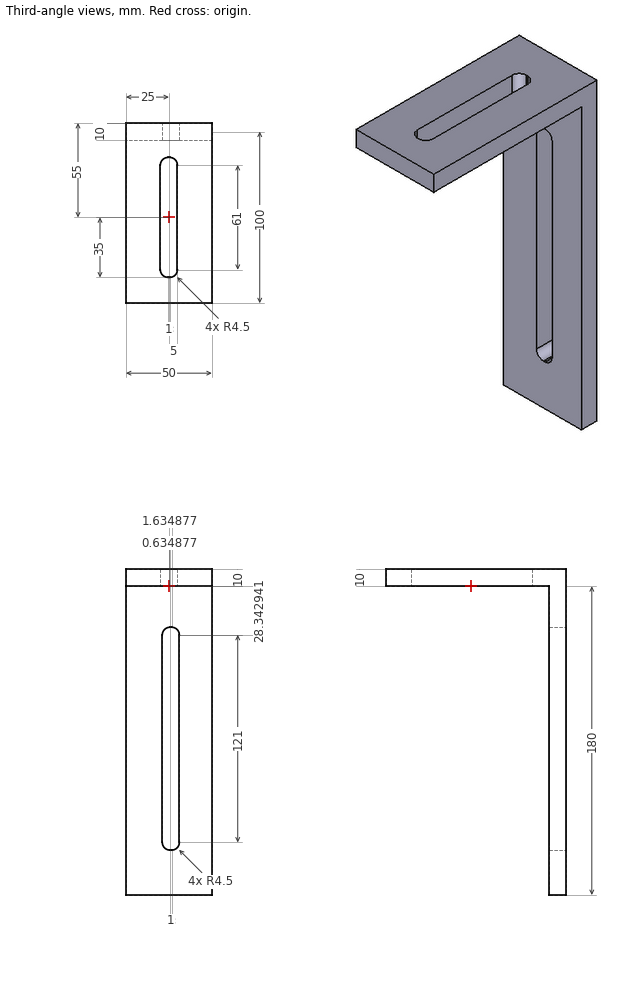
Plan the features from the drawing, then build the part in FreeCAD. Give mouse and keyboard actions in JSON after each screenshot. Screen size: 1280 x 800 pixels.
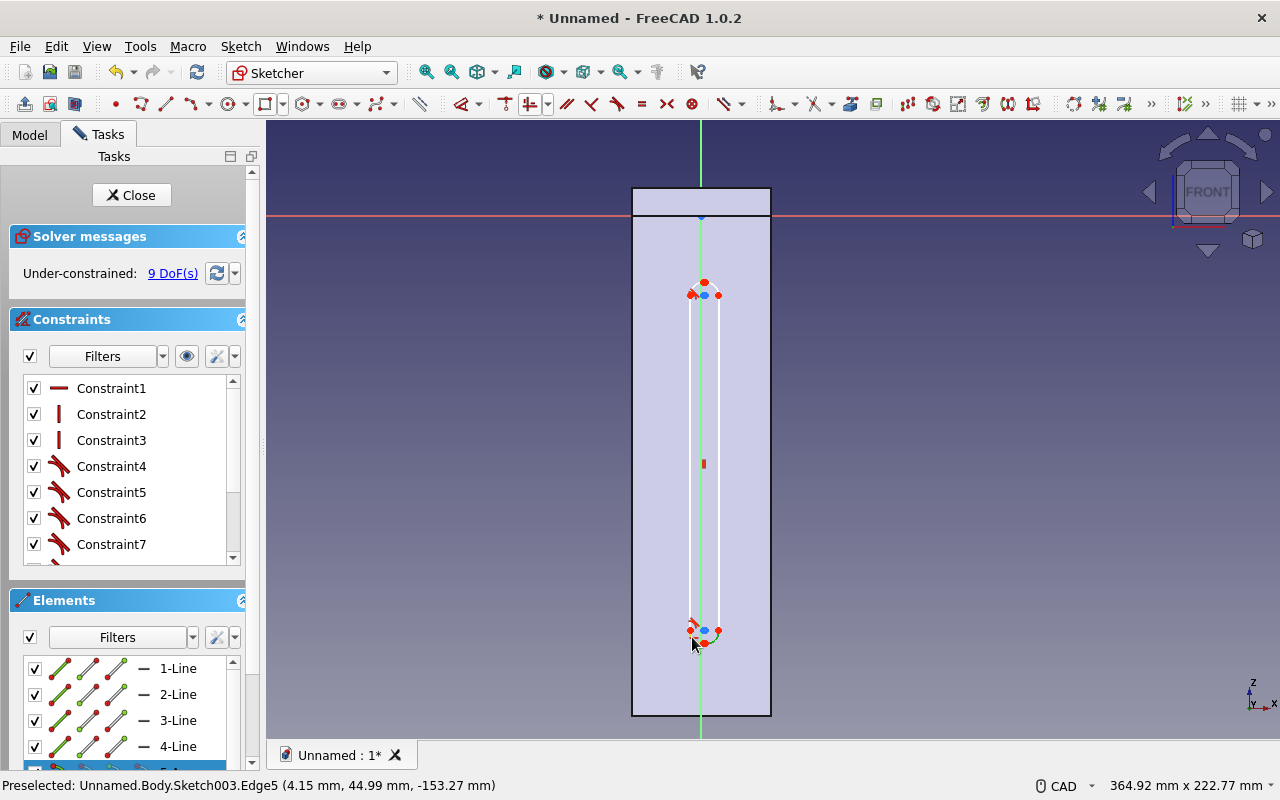
{"action": "scroll", "coordinate": [718, 290], "scroll_direction": "up", "scroll_amount": 5}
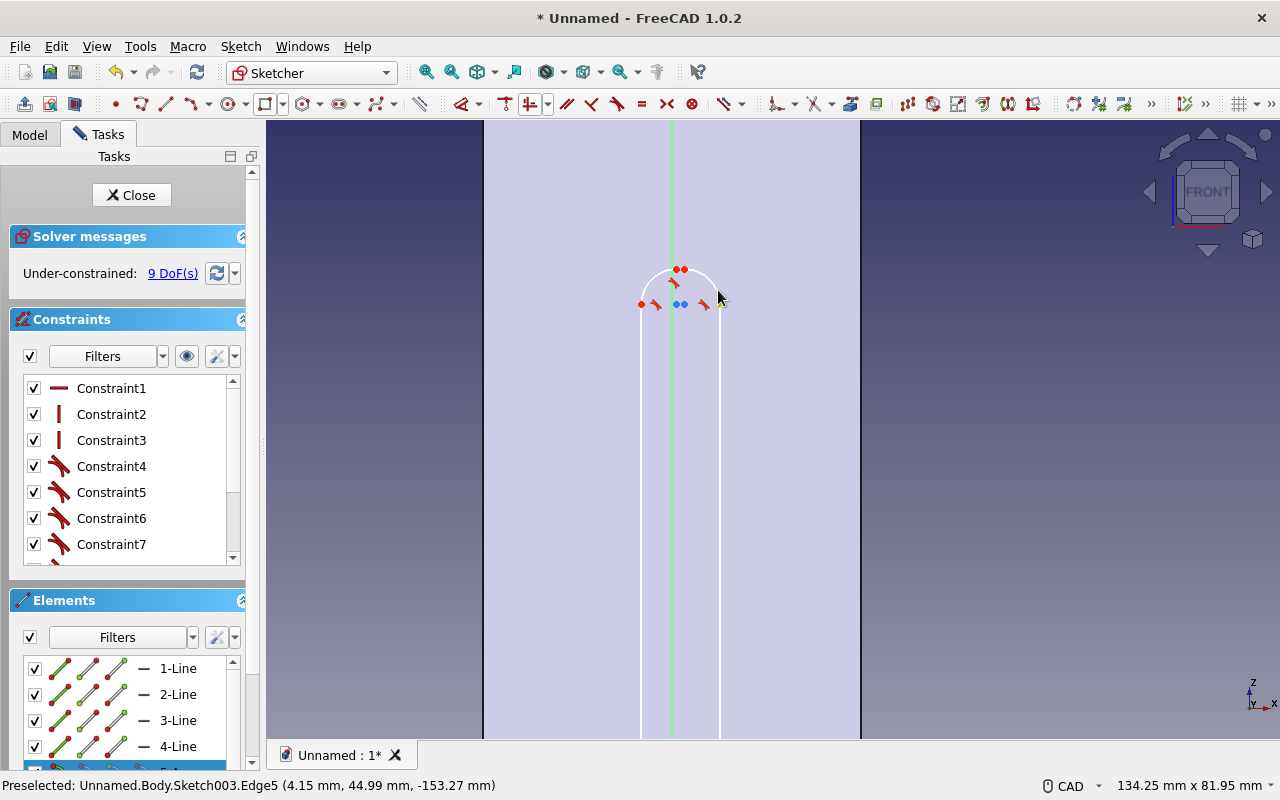
{"action": "left_click", "coordinate": [716, 288]}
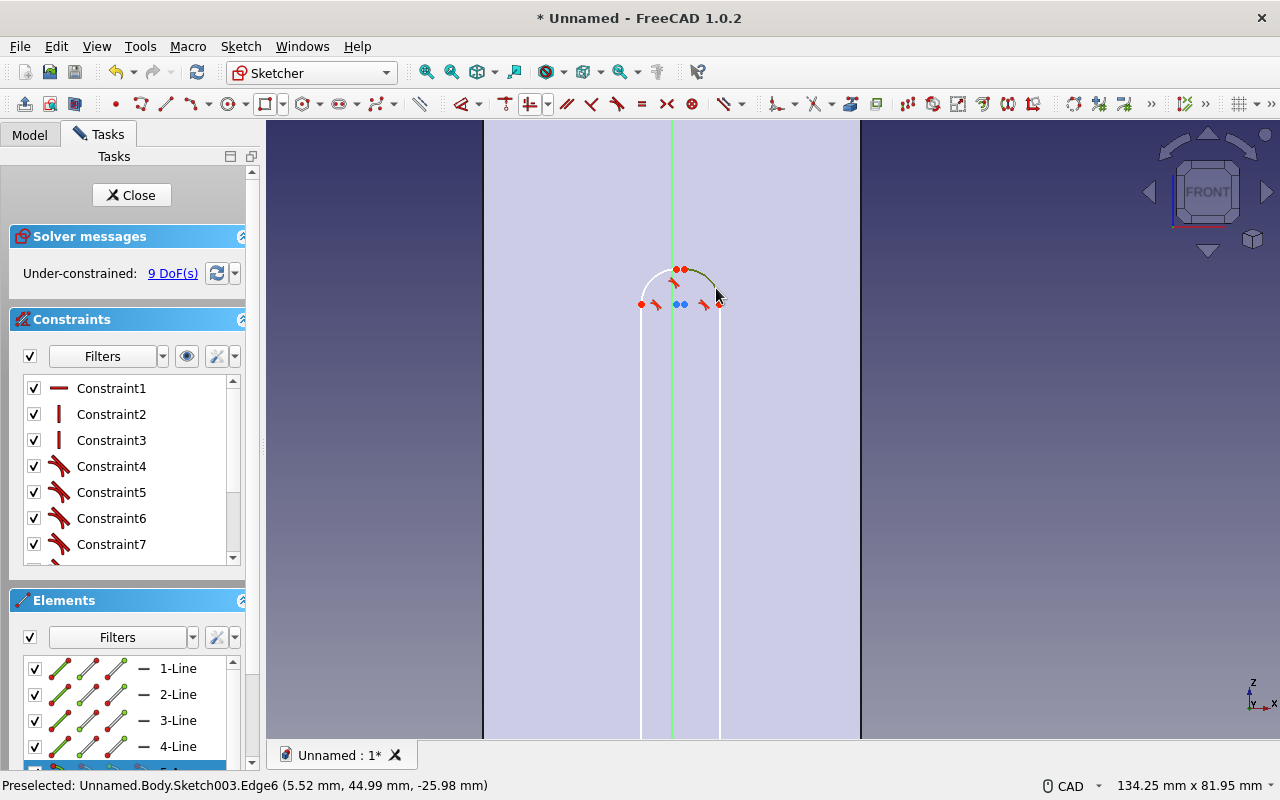
{"action": "scroll", "coordinate": [661, 273], "scroll_direction": "up", "scroll_amount": 2}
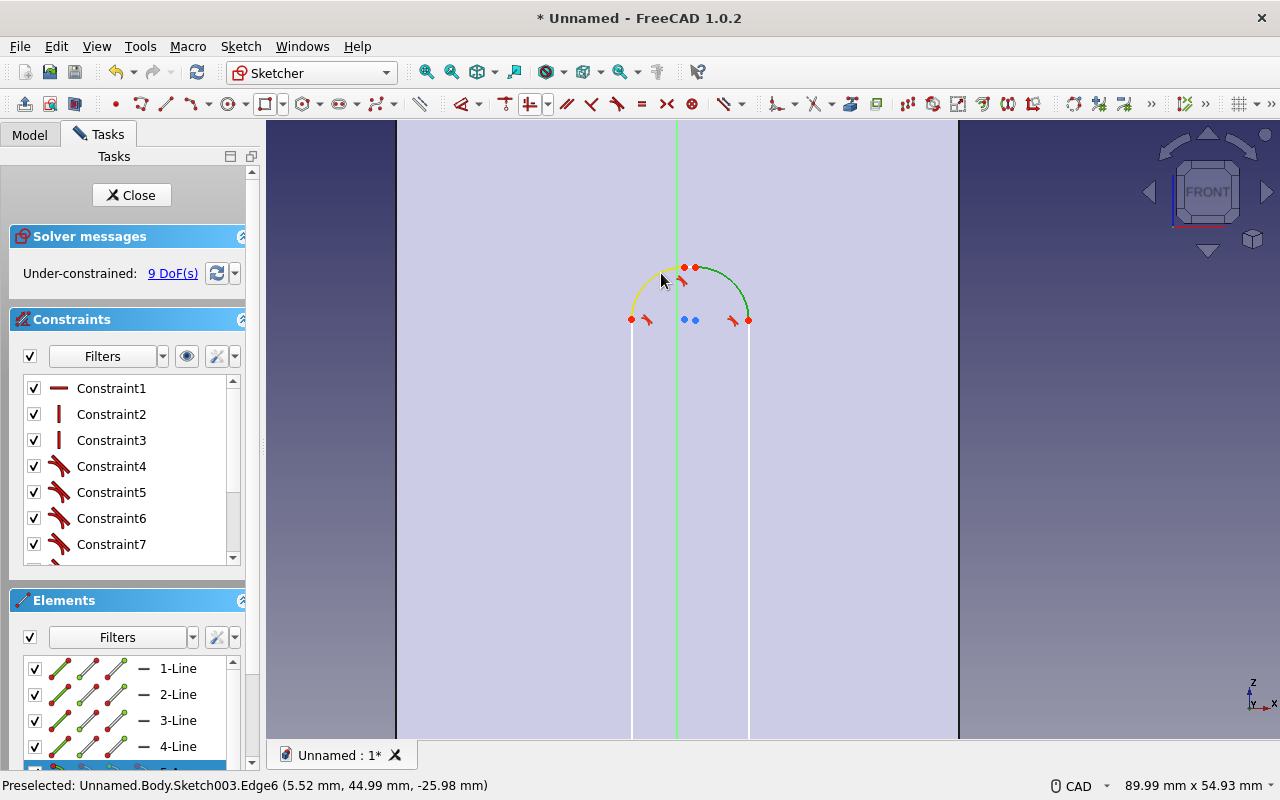
{"action": "left_click", "coordinate": [660, 273]}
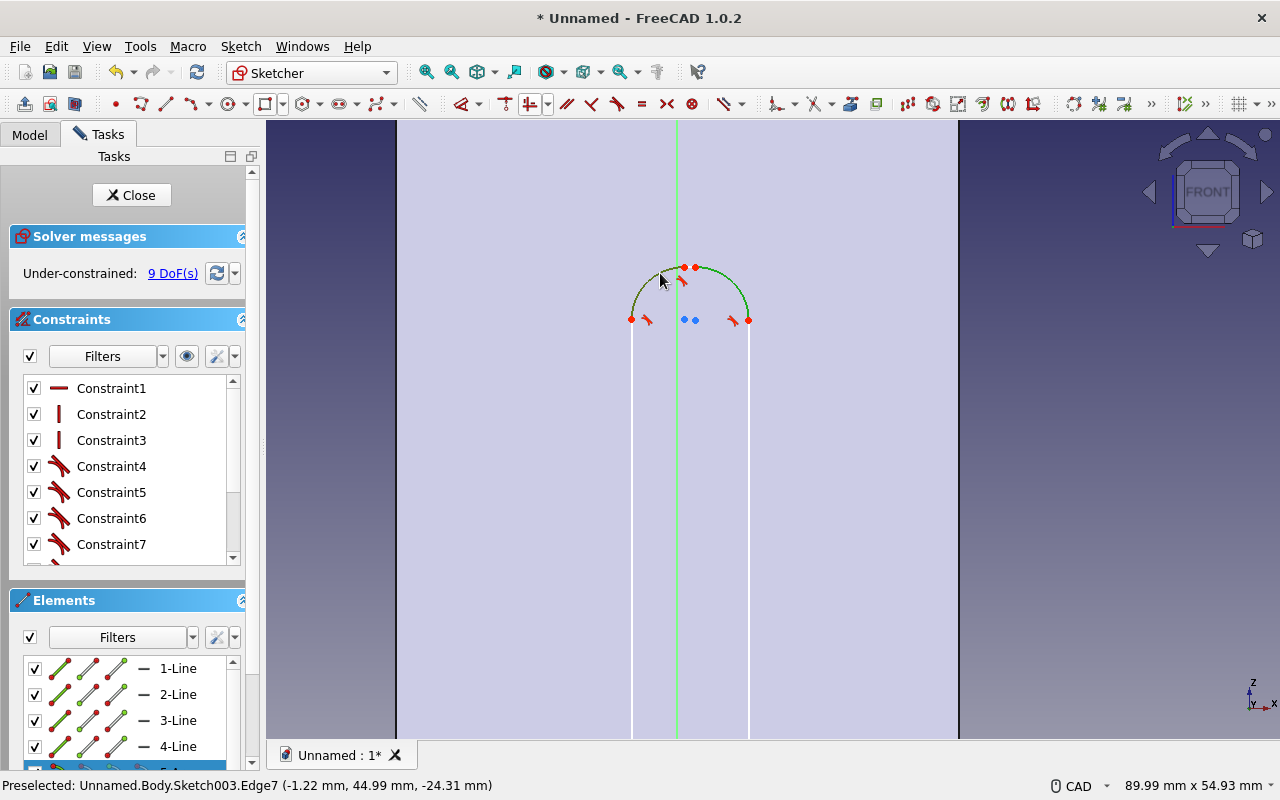
{"action": "scroll", "coordinate": [709, 287], "scroll_direction": "down", "scroll_amount": 7}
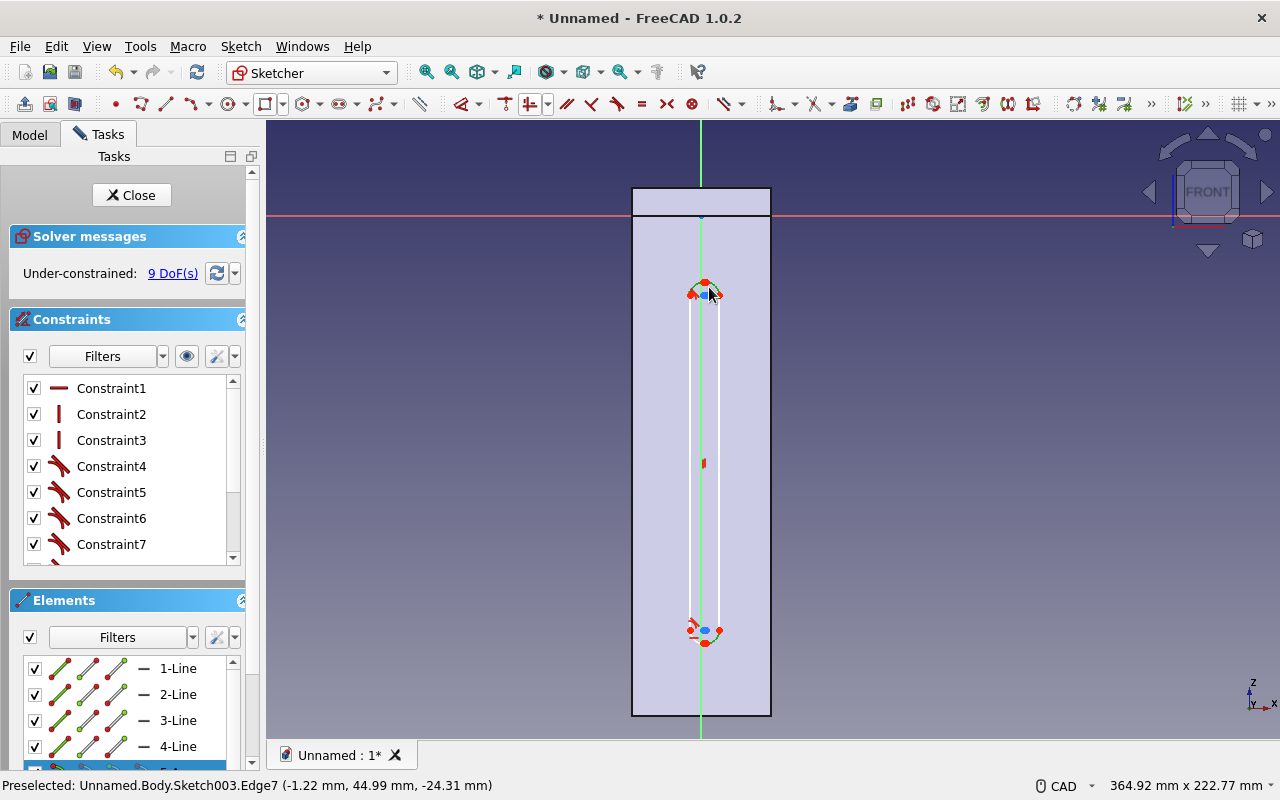
{"action": "scroll", "coordinate": [692, 636], "scroll_direction": "up", "scroll_amount": 4}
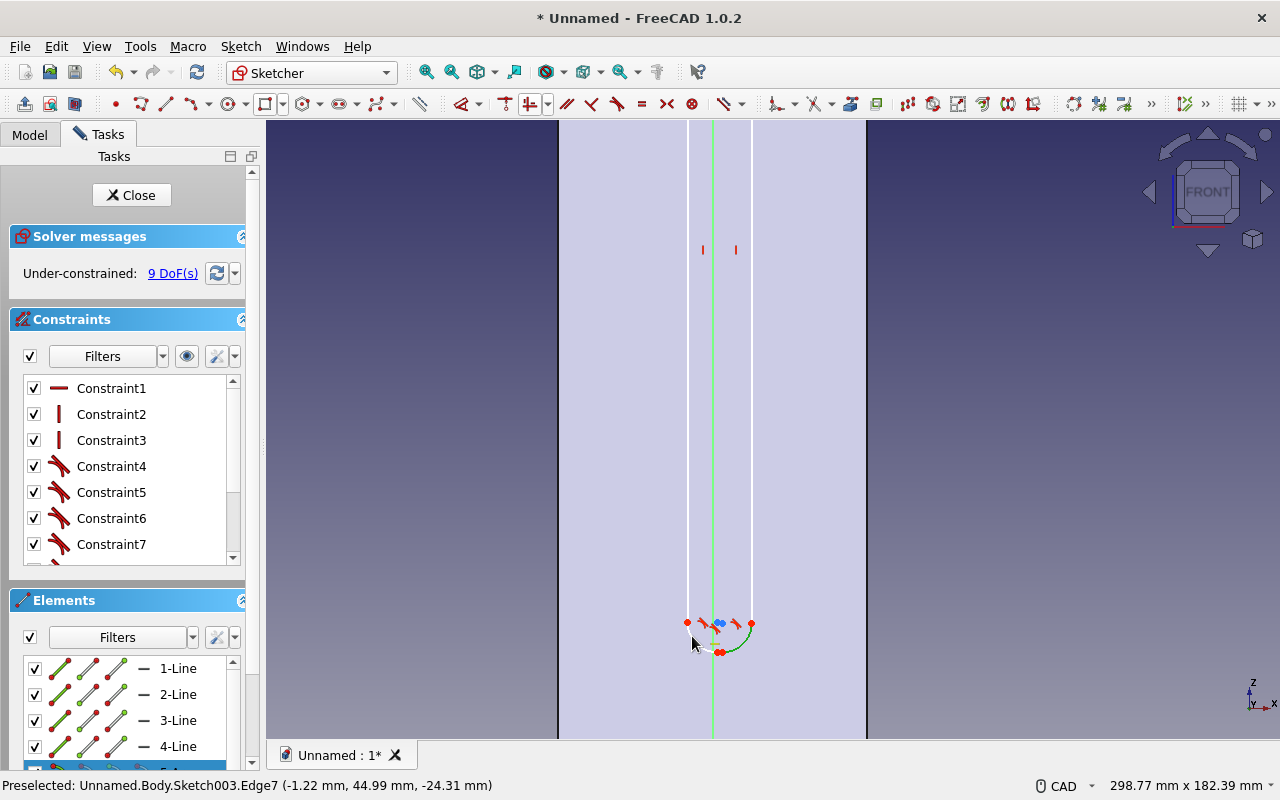
{"action": "left_click", "coordinate": [691, 636]}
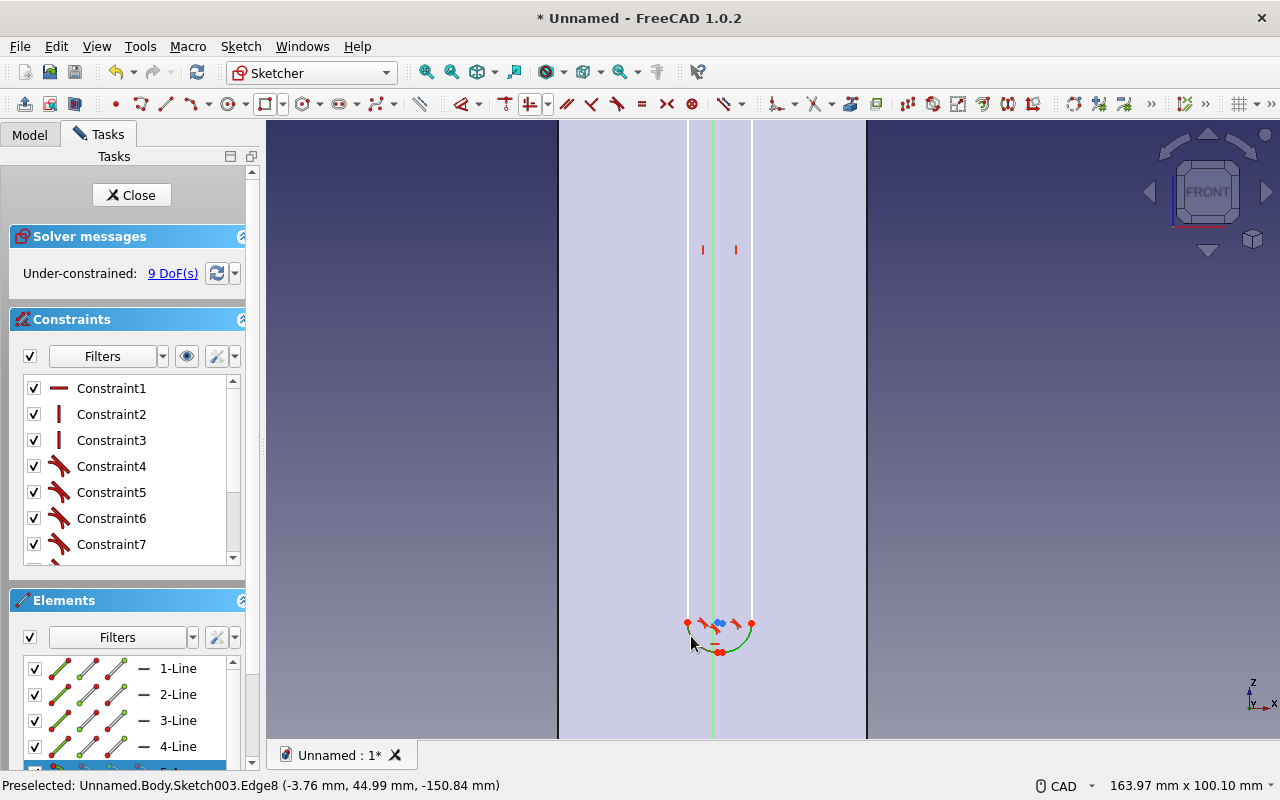
{"action": "left_click", "coordinate": [642, 104]}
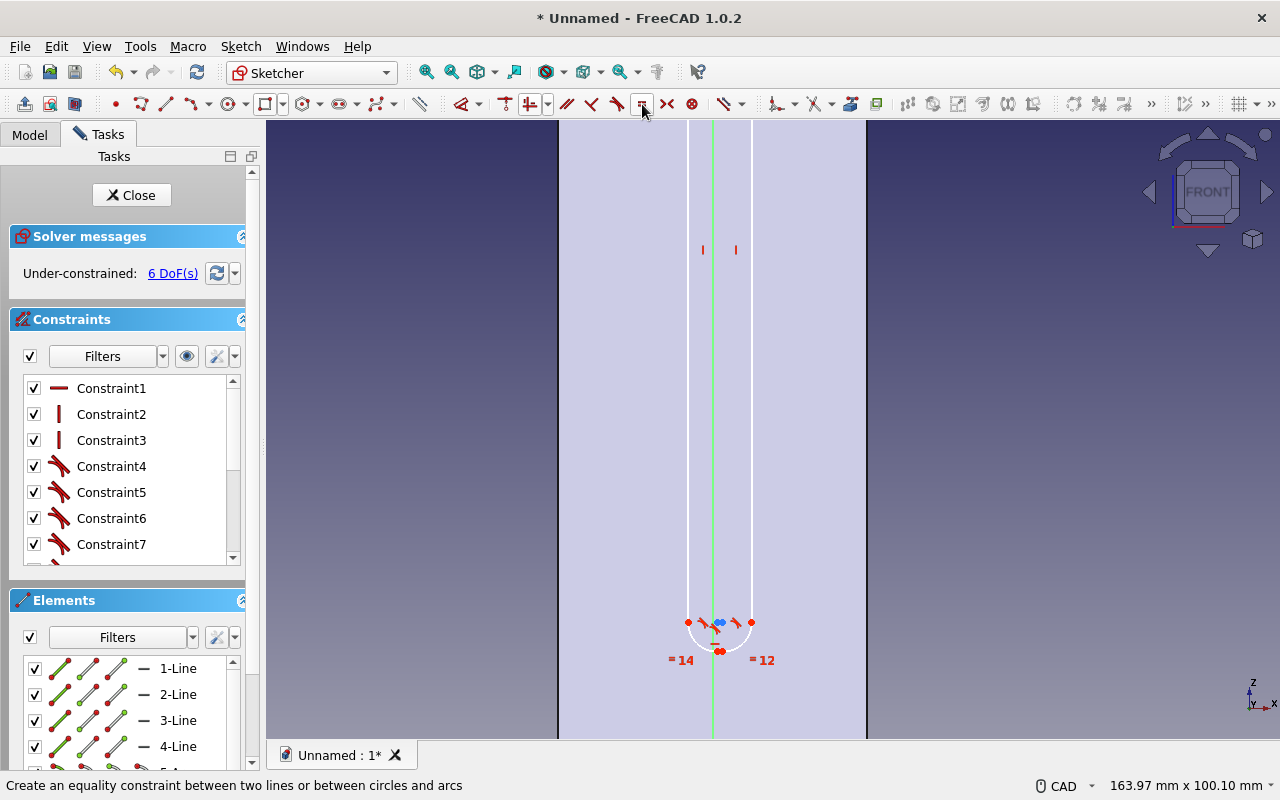
{"action": "left_click", "coordinate": [460, 104]}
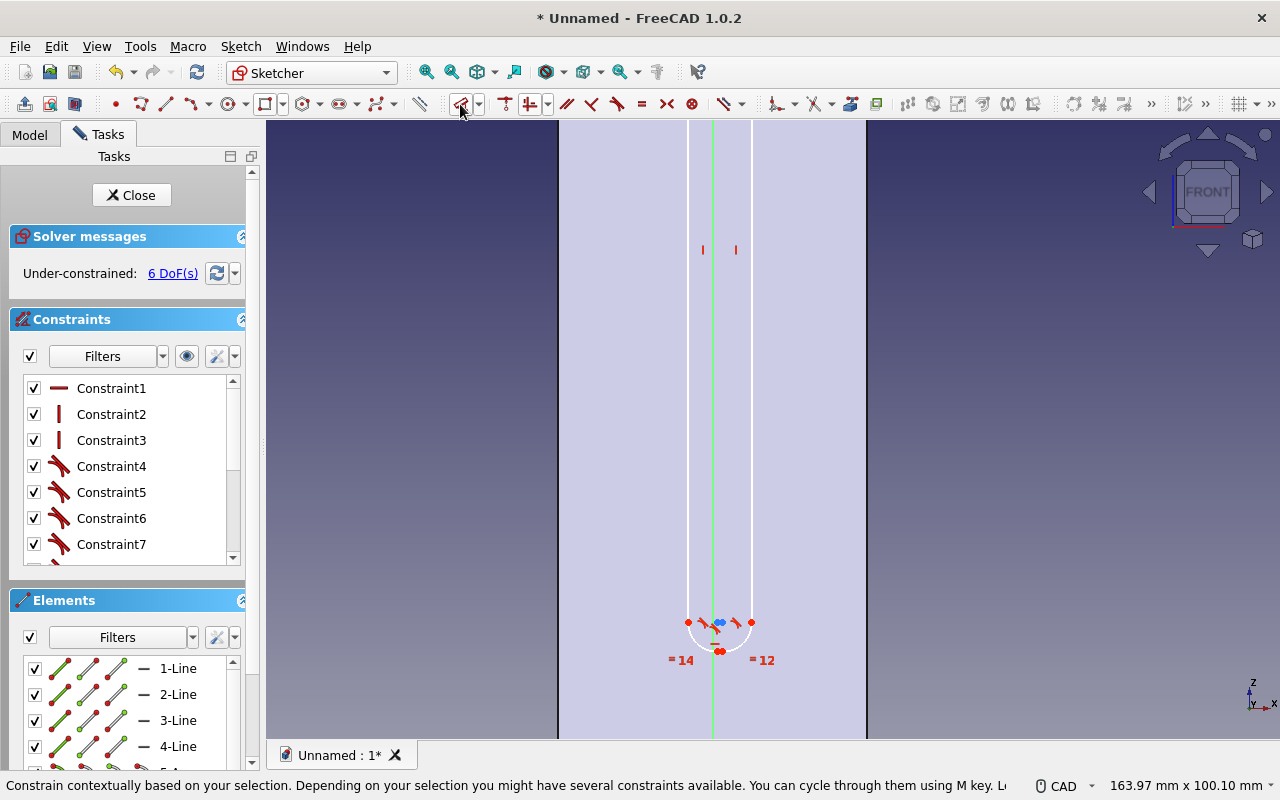
{"action": "scroll", "coordinate": [736, 648], "scroll_direction": "up", "scroll_amount": 2}